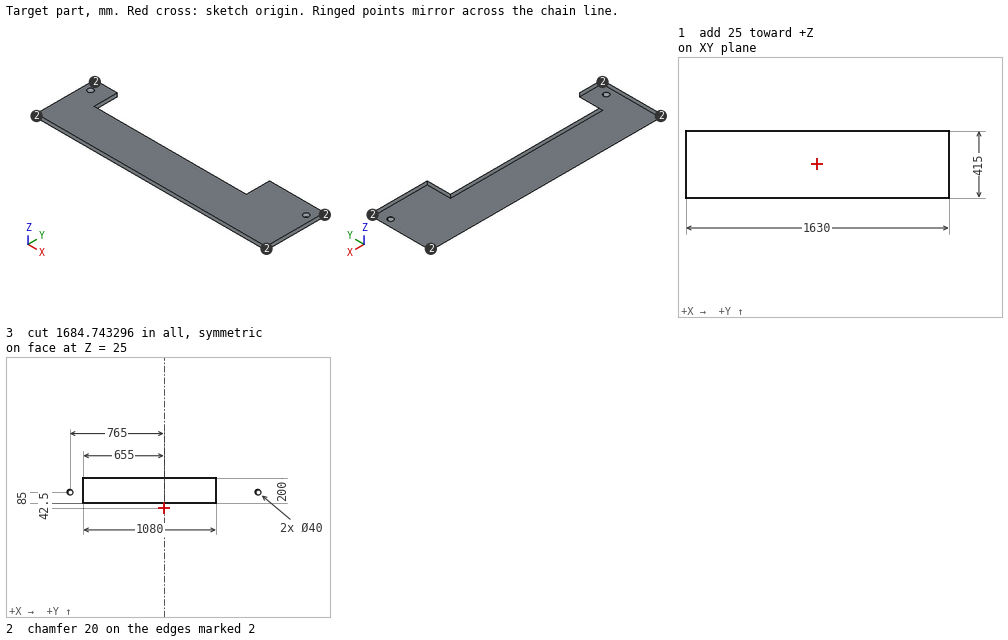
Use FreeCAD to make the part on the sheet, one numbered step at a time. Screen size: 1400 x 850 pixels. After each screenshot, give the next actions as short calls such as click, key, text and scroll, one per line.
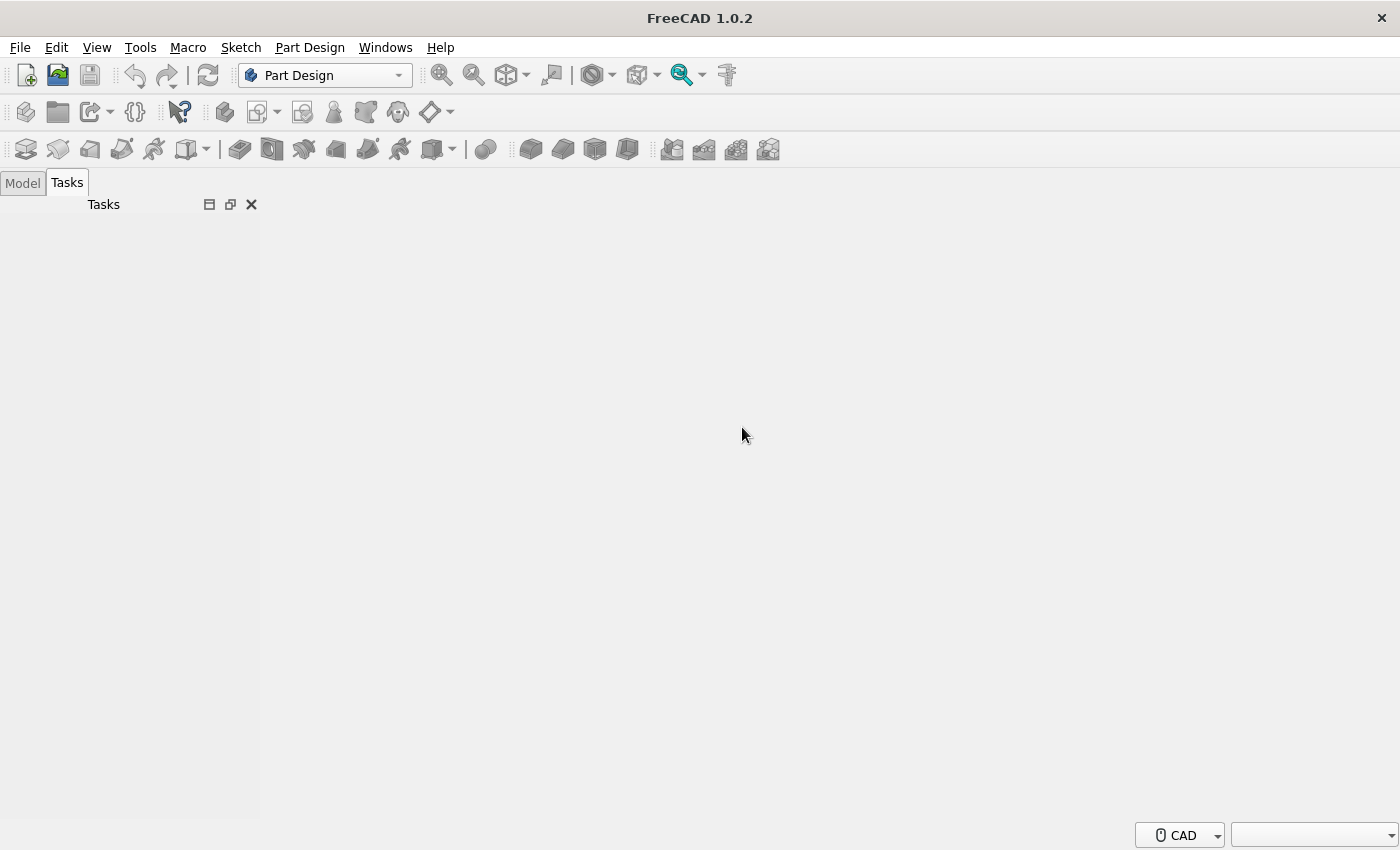
click(26, 76)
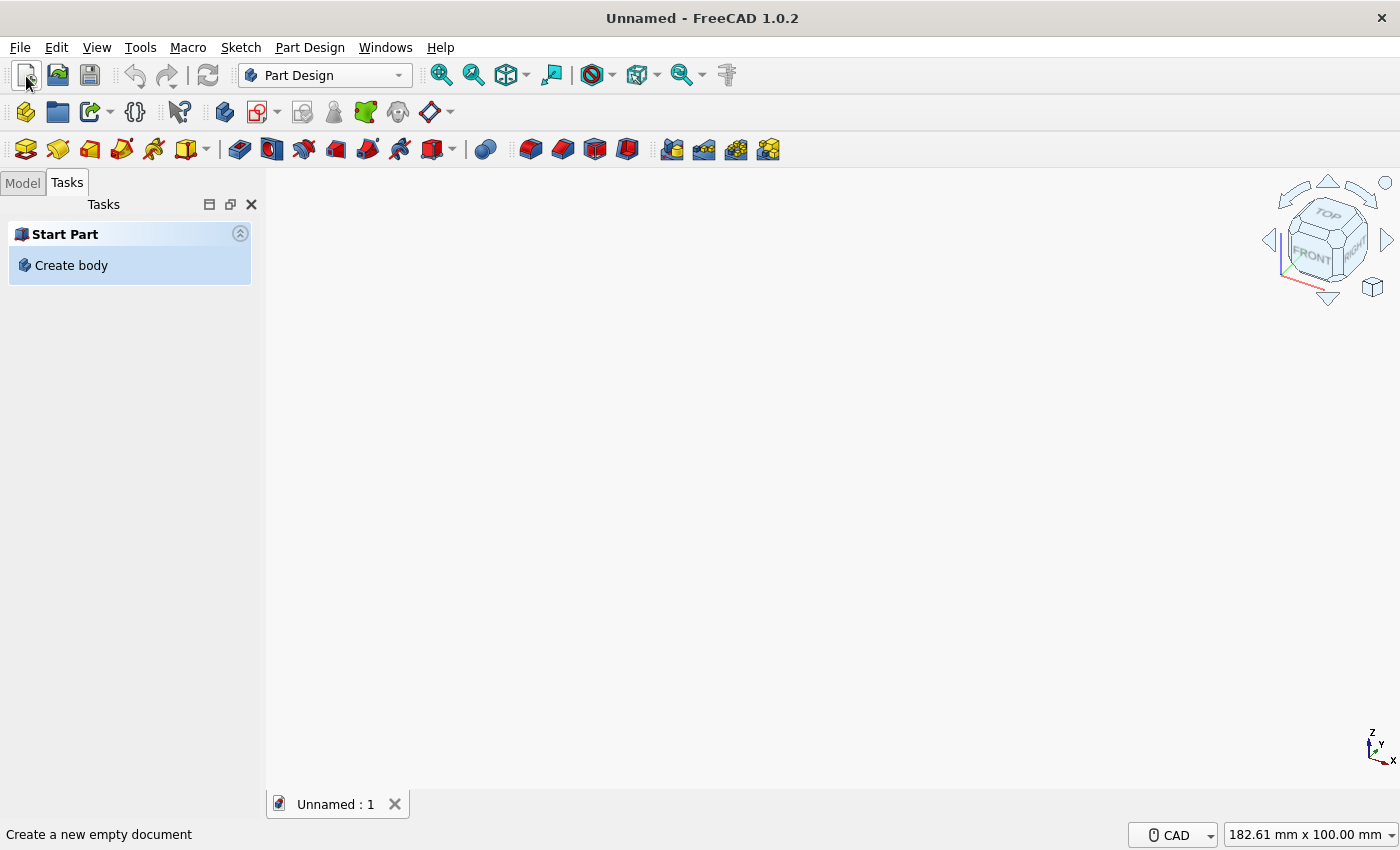
click(258, 112)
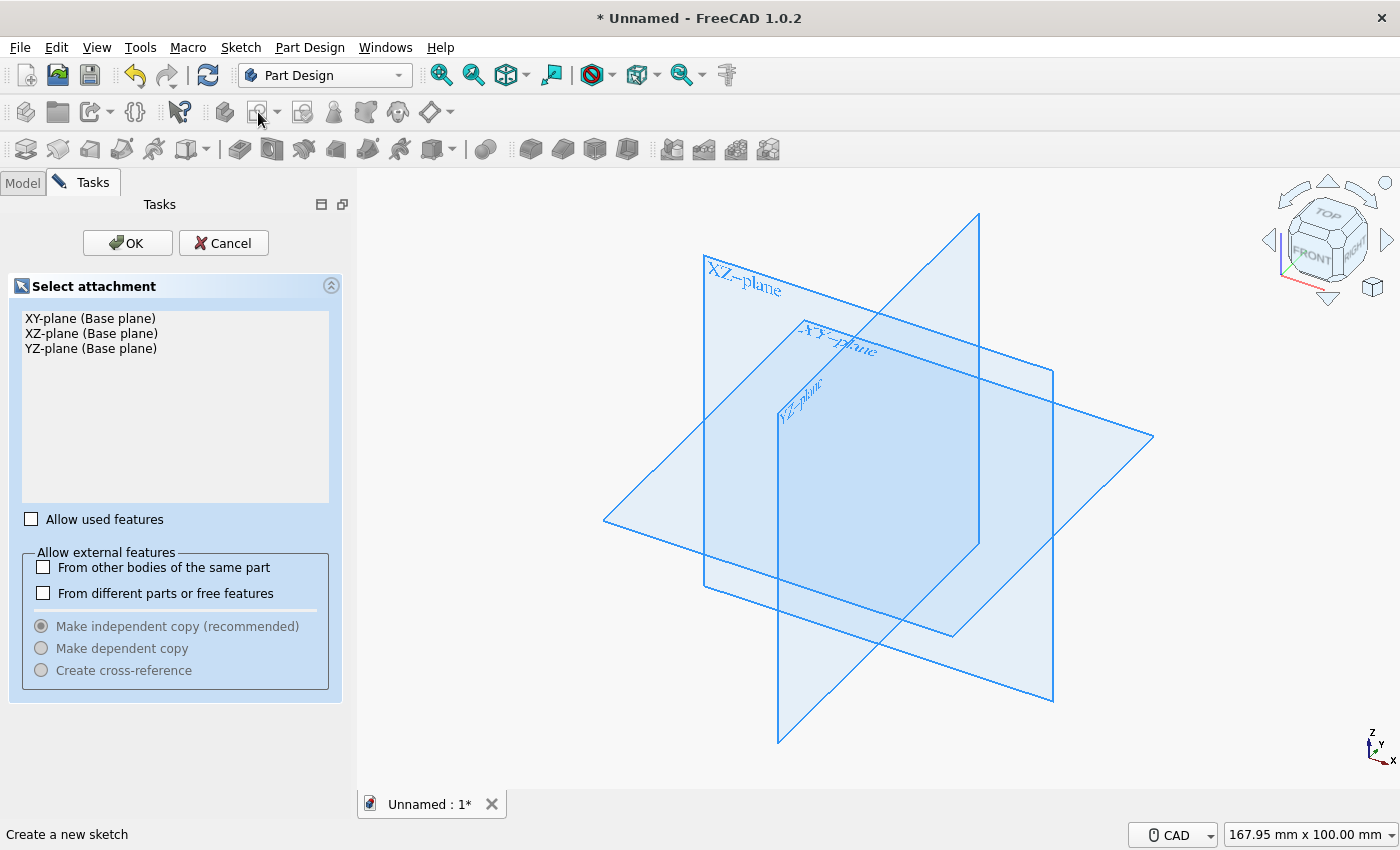
click(82, 318)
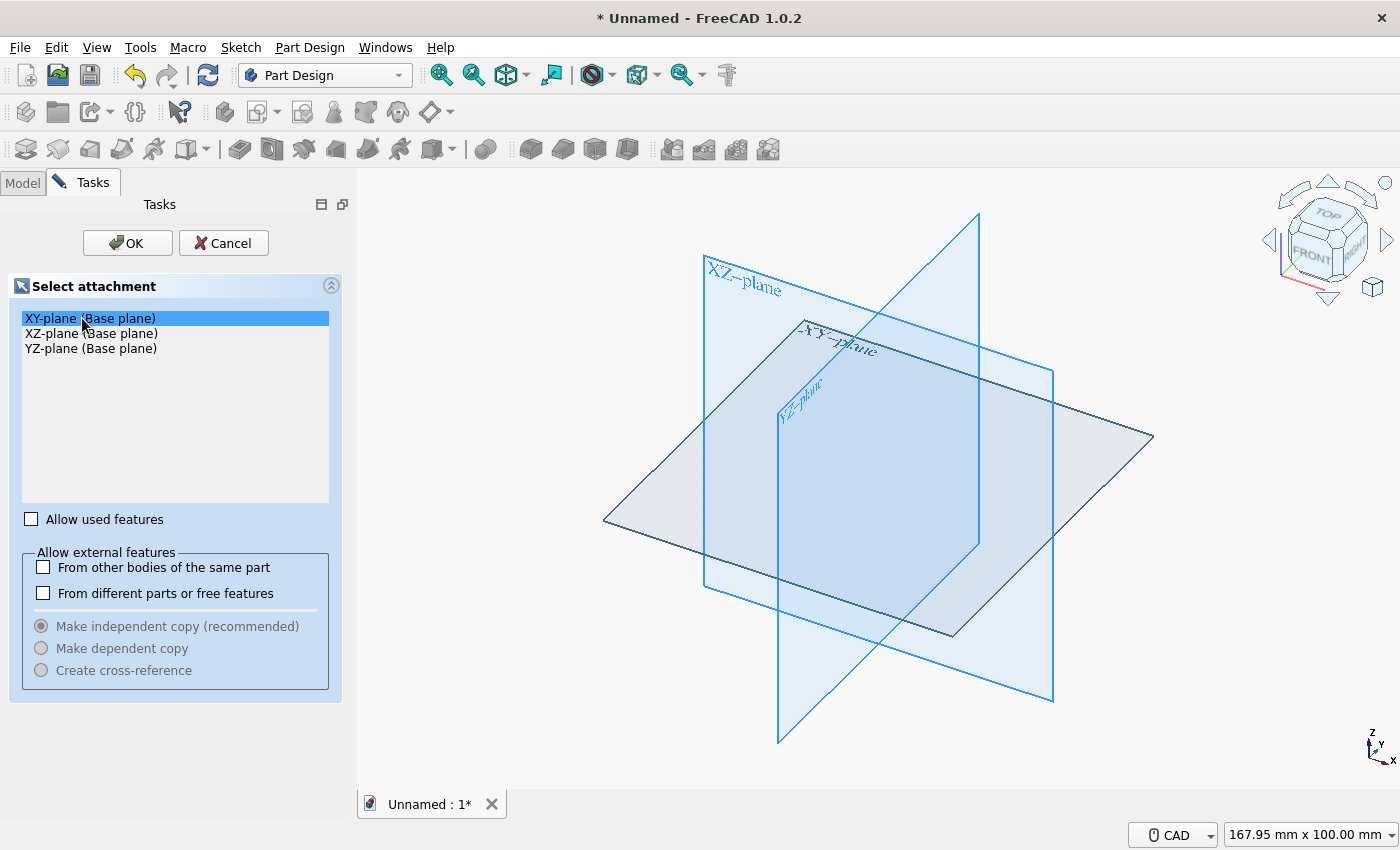
click(128, 243)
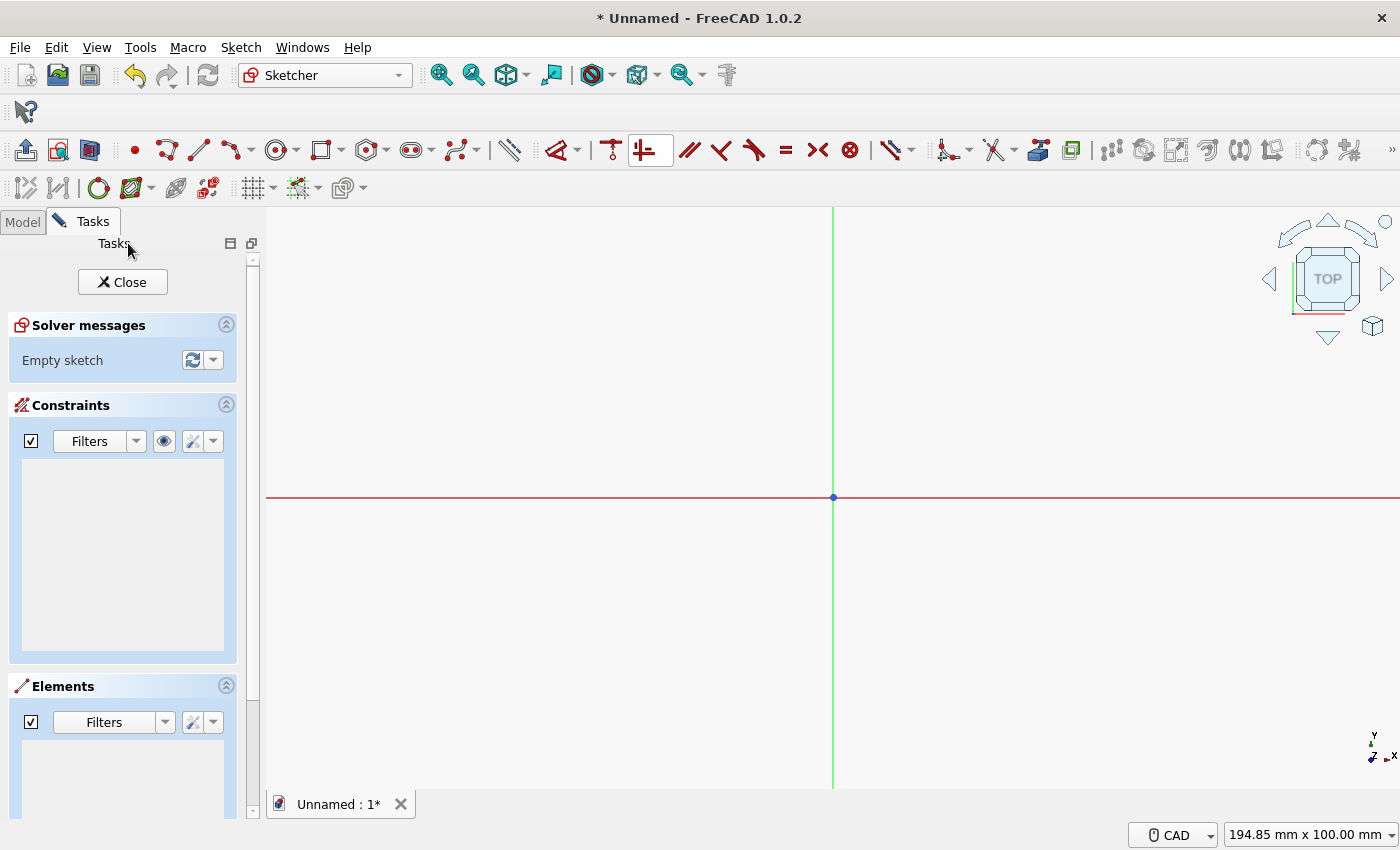
scroll(759, 498, down, 13)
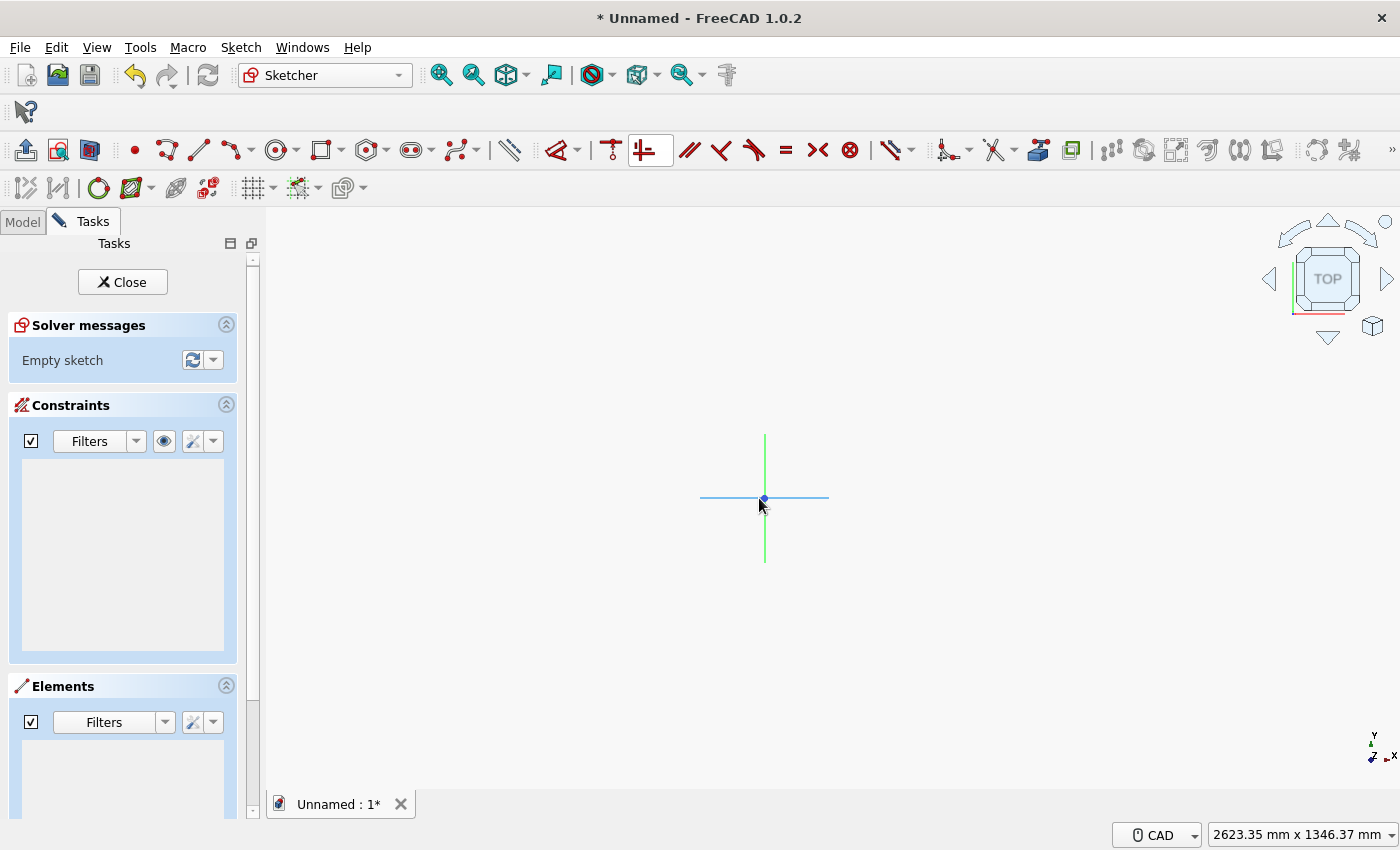
click(344, 150)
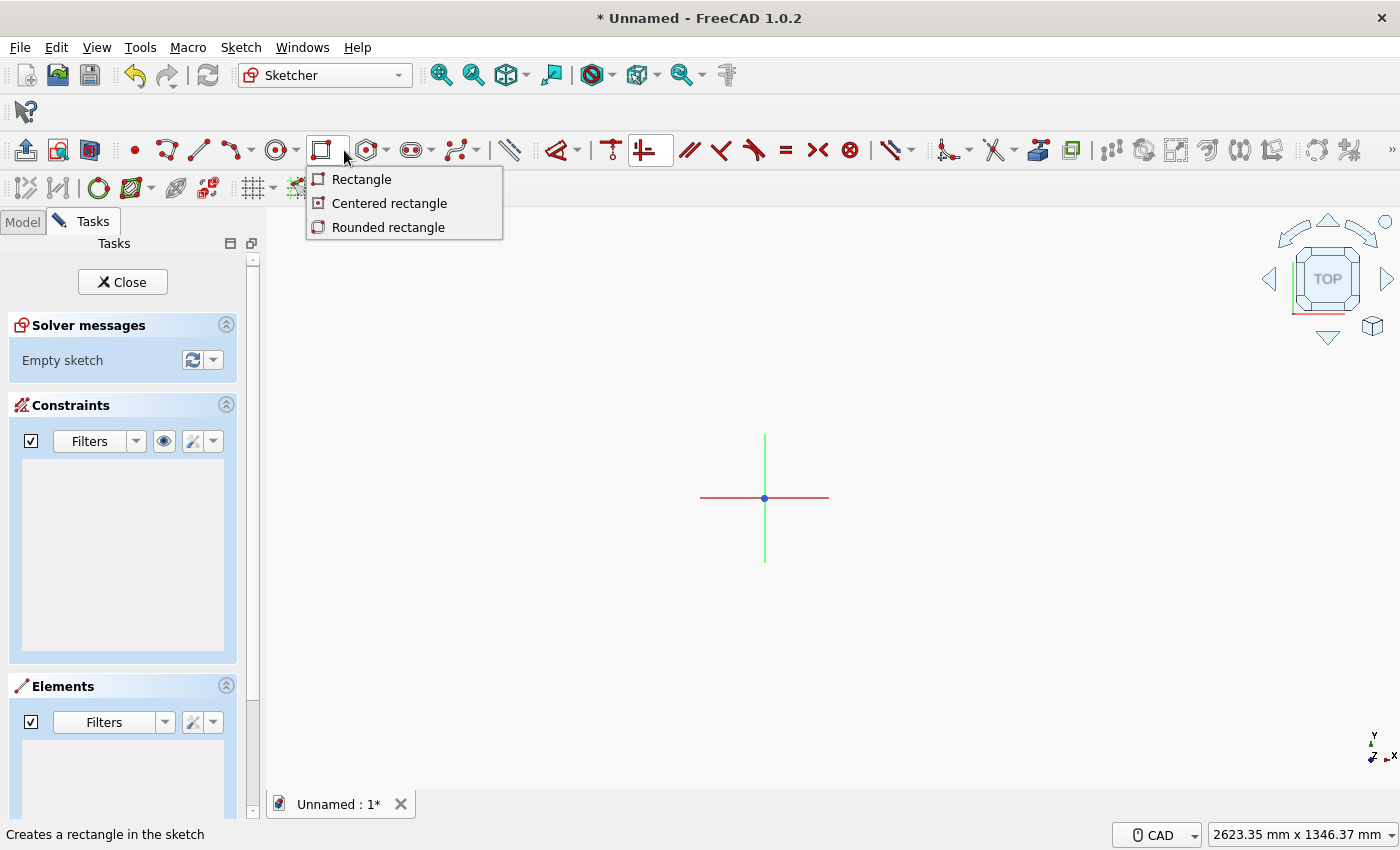
click(404, 203)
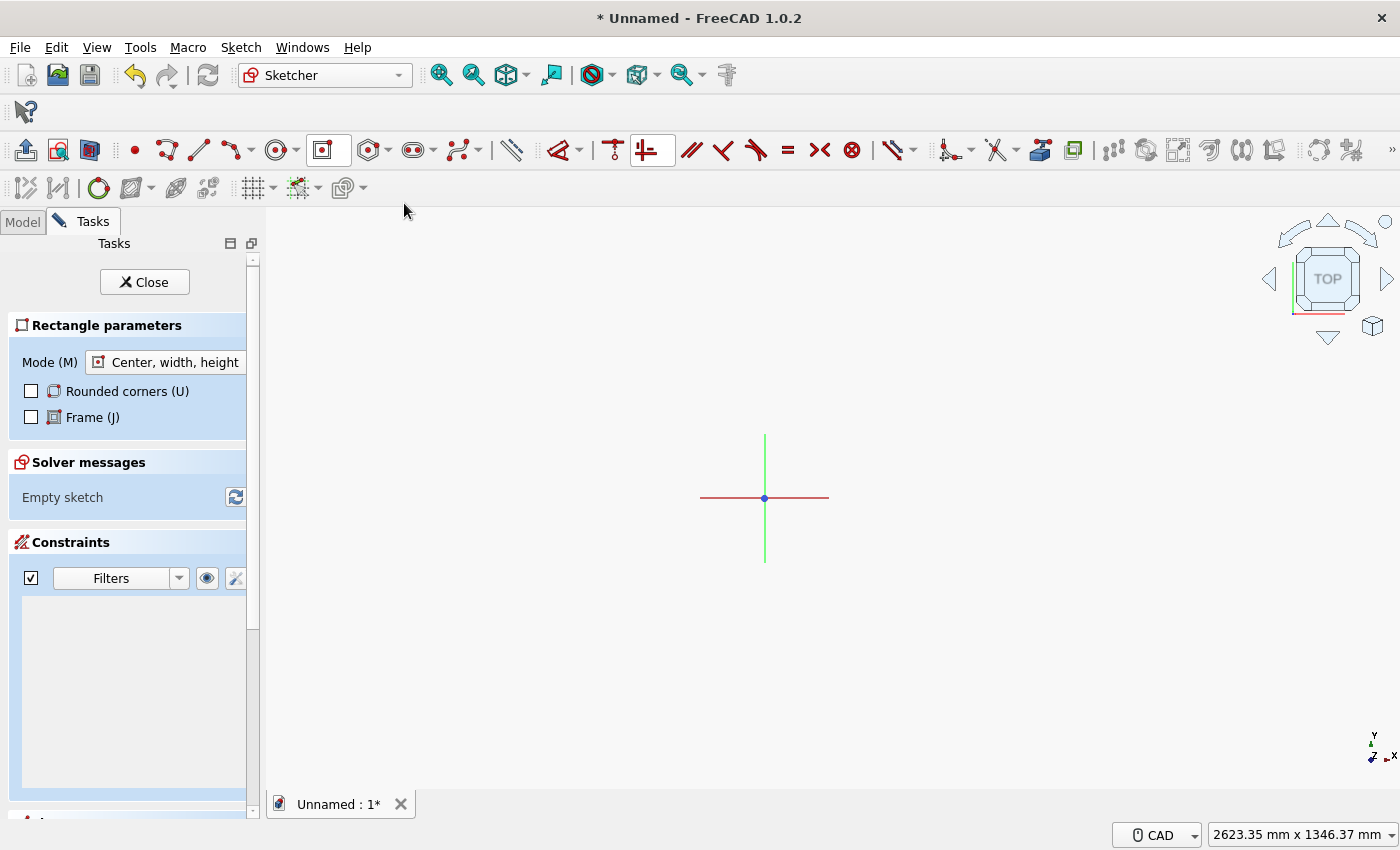
click(765, 498)
move(1117, 409)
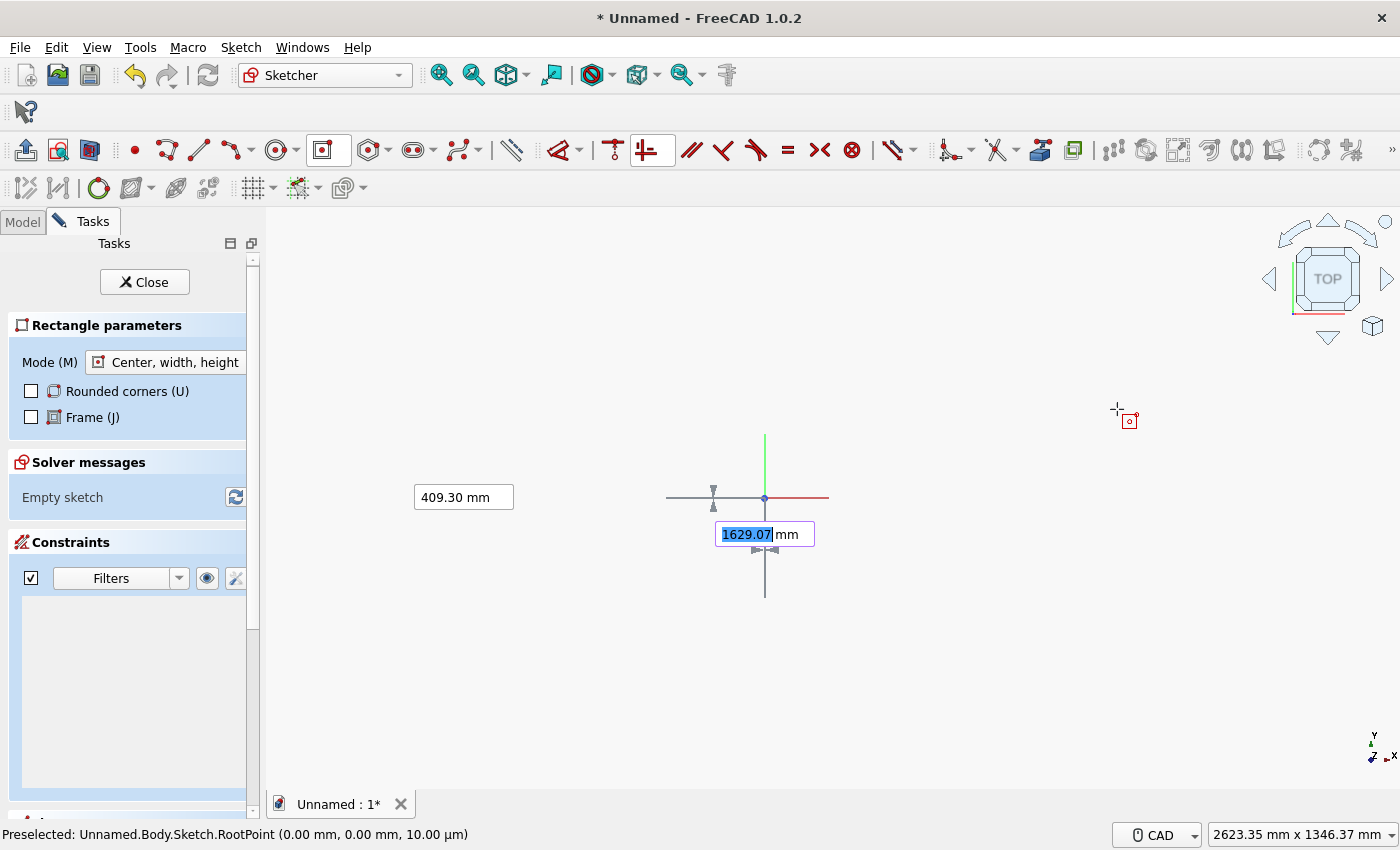
text(1630)
key(Tab)
text(415)
key(Return)
key(Escape)